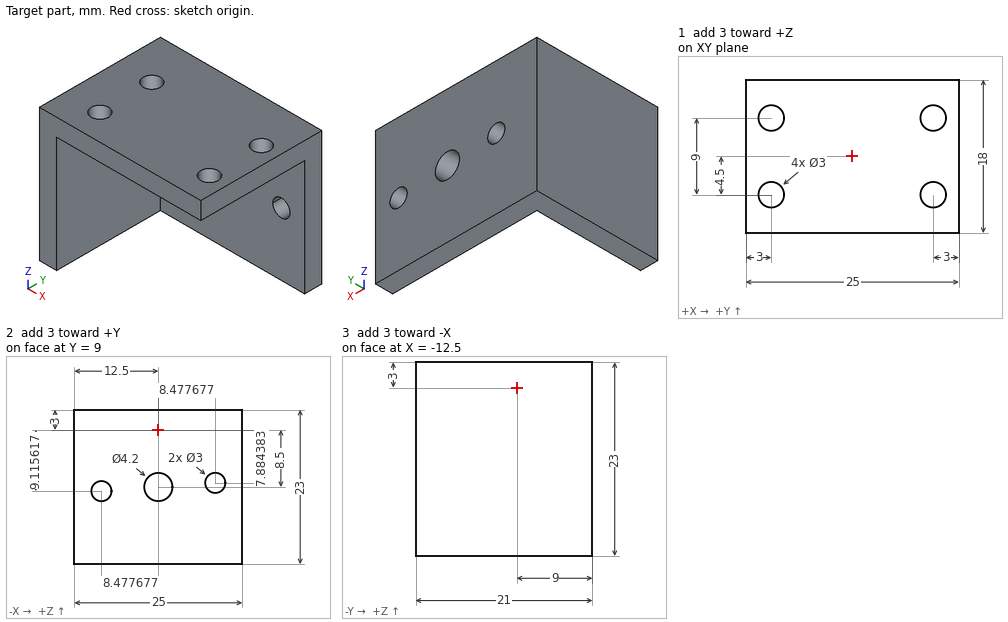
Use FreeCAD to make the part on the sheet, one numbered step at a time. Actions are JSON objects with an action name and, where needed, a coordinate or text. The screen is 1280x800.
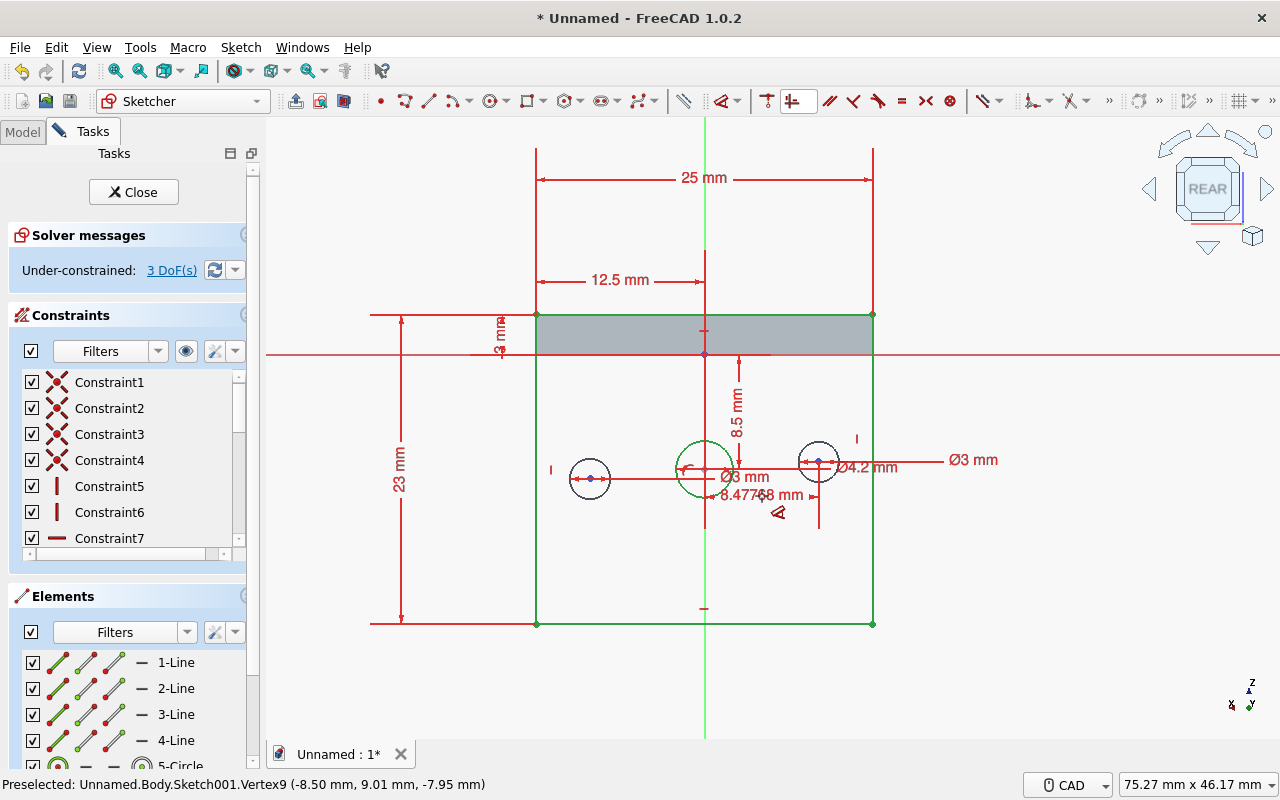
{"action": "left_click", "coordinate": [819, 462]}
{"action": "left_click", "coordinate": [853, 408]}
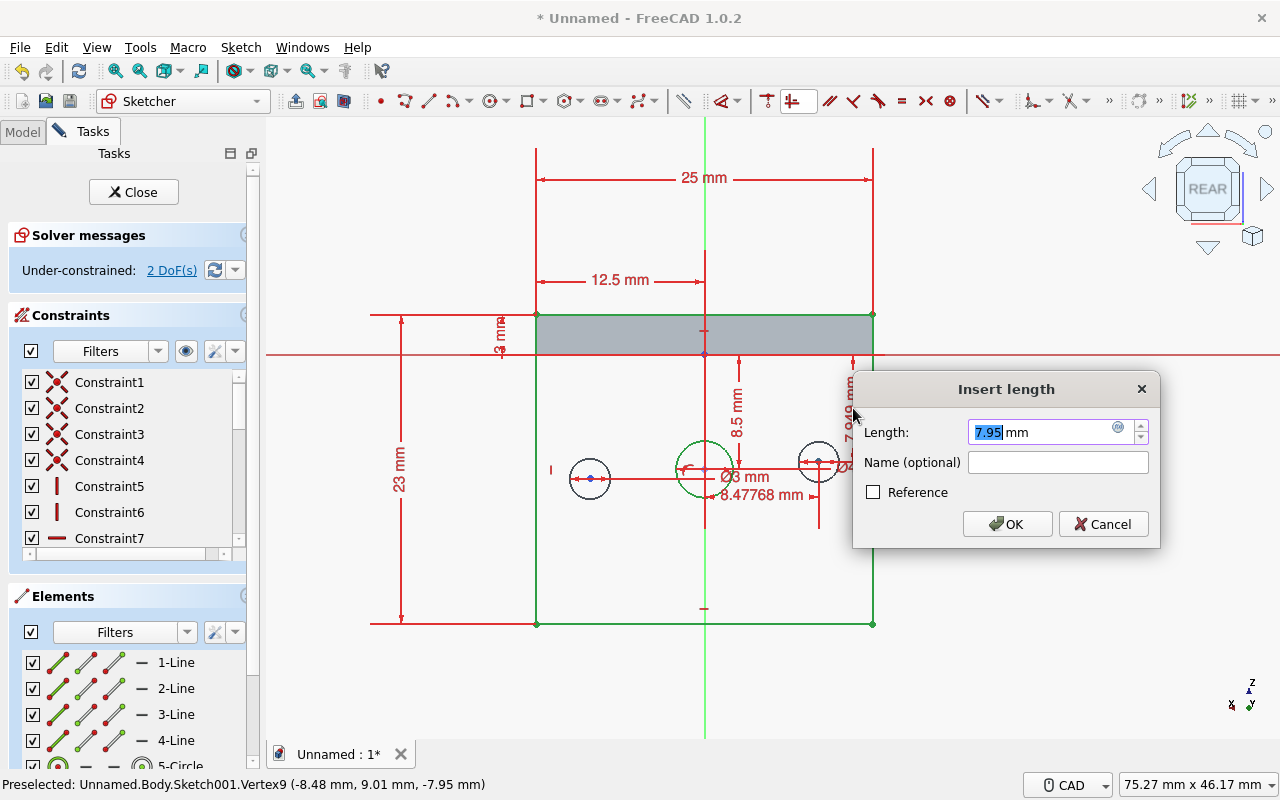
{"action": "type", "text": "7.884383"}
{"action": "key", "text": "Return"}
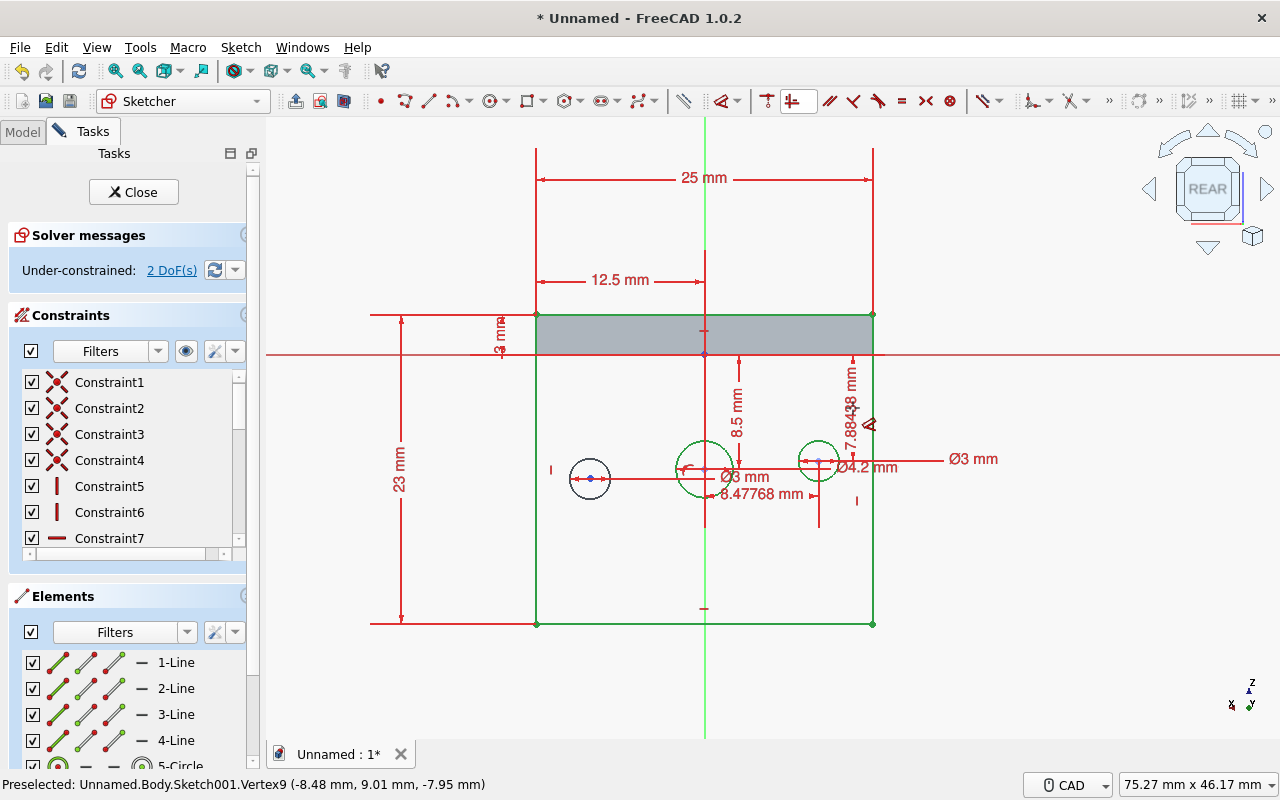
{"action": "left_click", "coordinate": [590, 479]}
{"action": "left_click", "coordinate": [647, 513]}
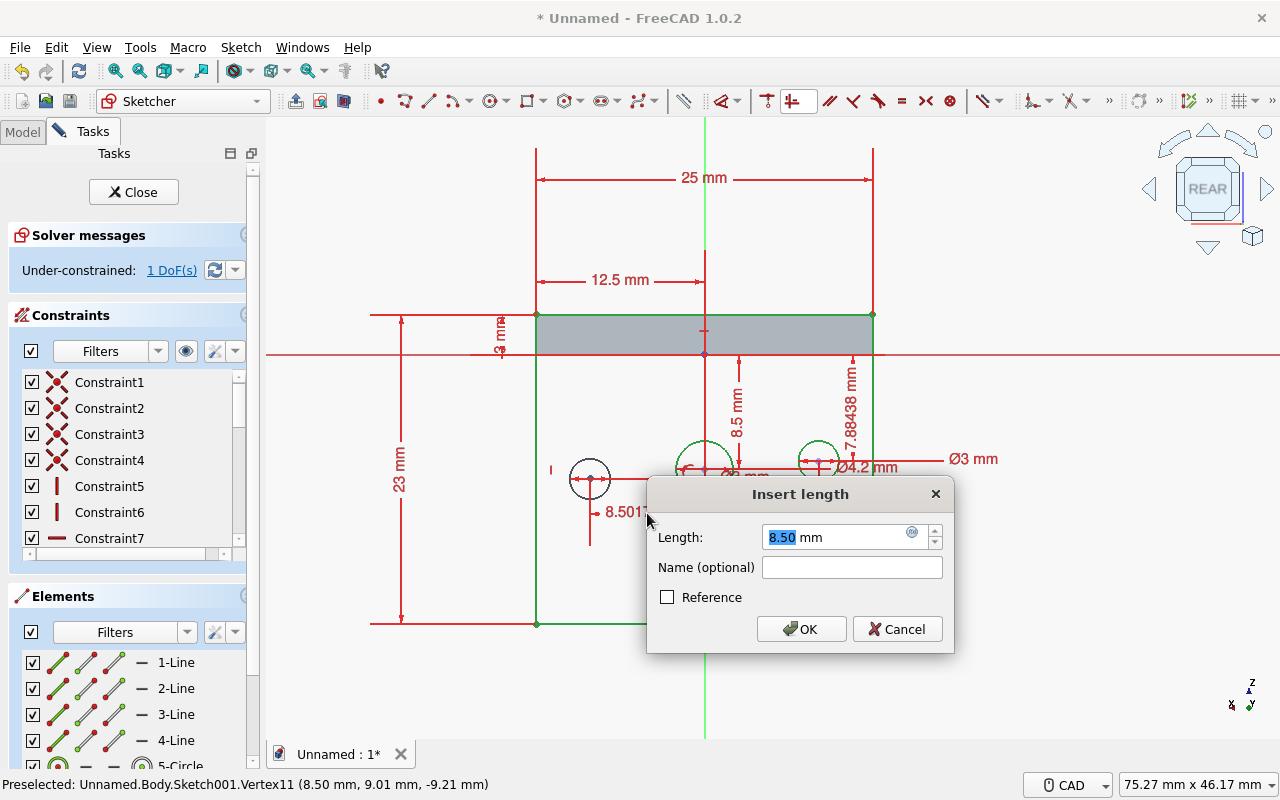
{"action": "type", "text": "8.477677"}
{"action": "key", "text": "Return"}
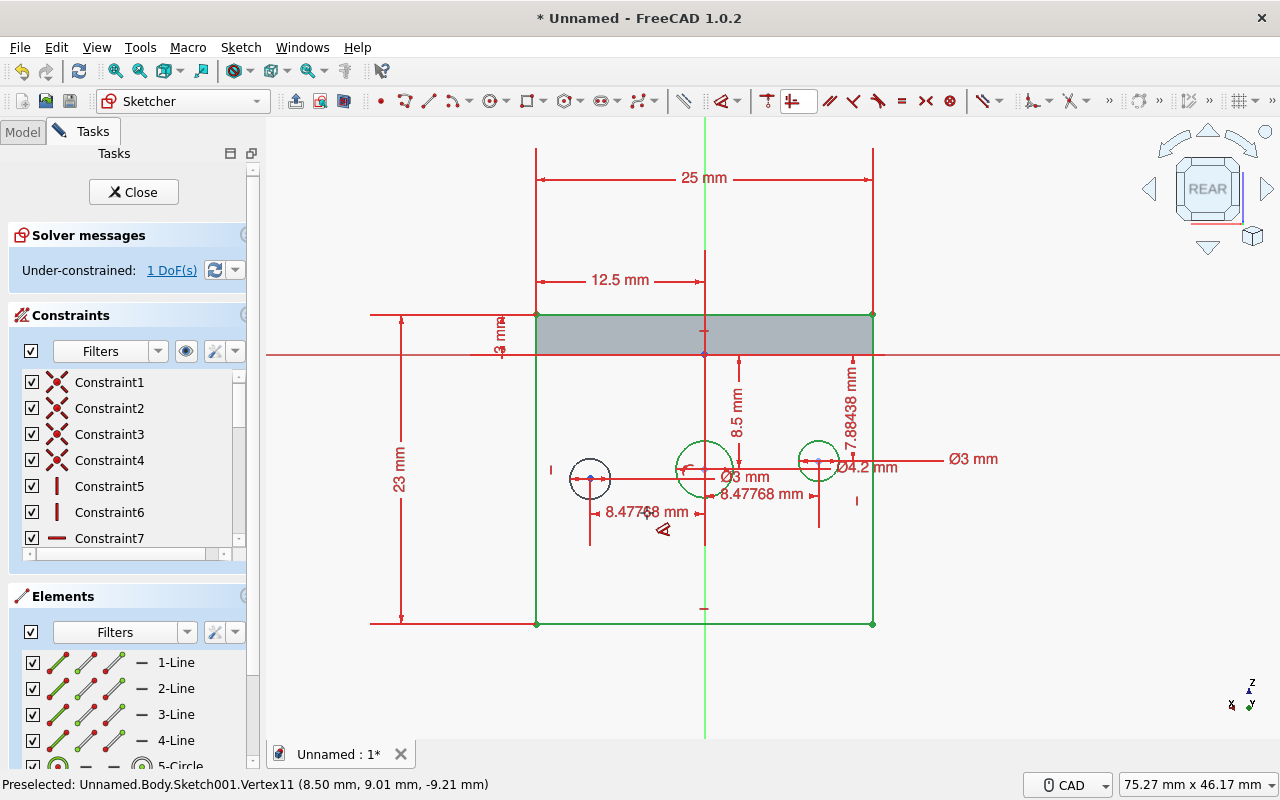
{"action": "left_click", "coordinate": [590, 479]}
{"action": "left_click", "coordinate": [556, 417]}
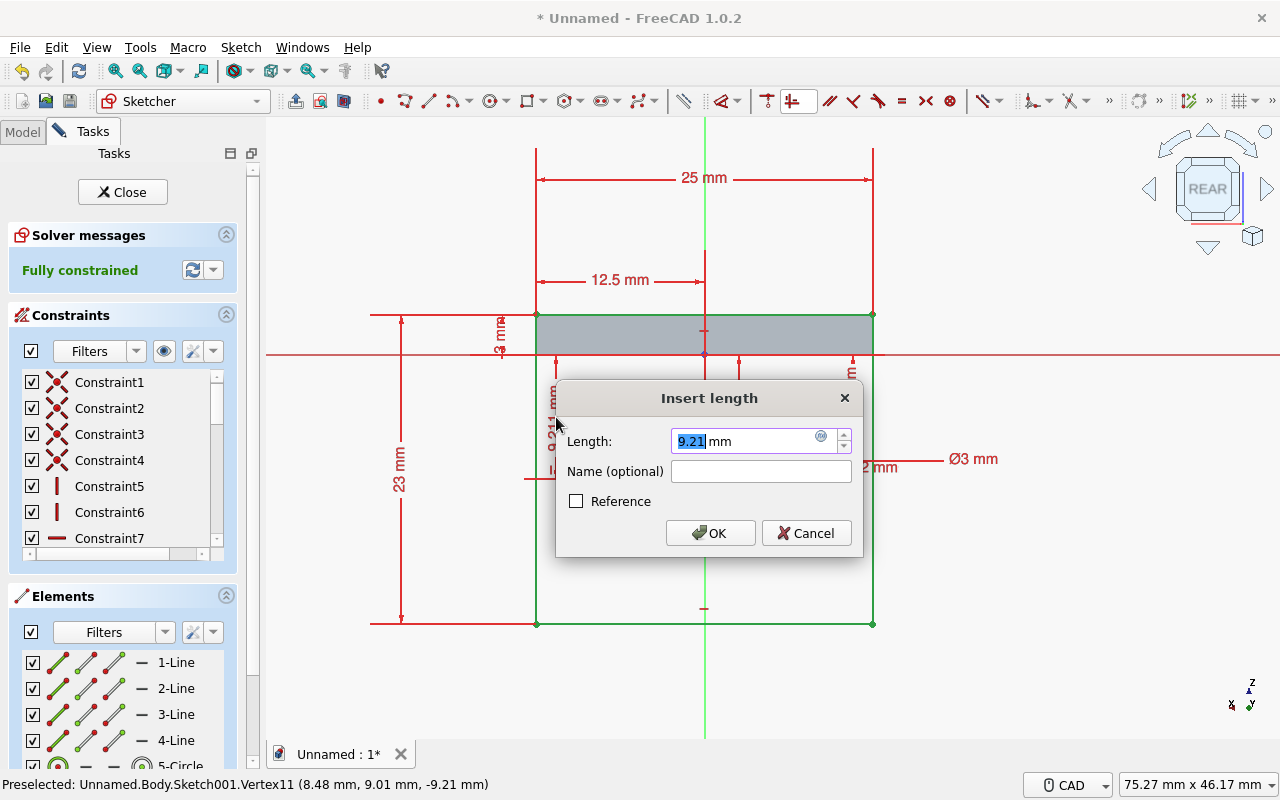
{"action": "type", "text": "9.115617"}
{"action": "key", "text": "Return"}
{"action": "key", "text": "Escape"}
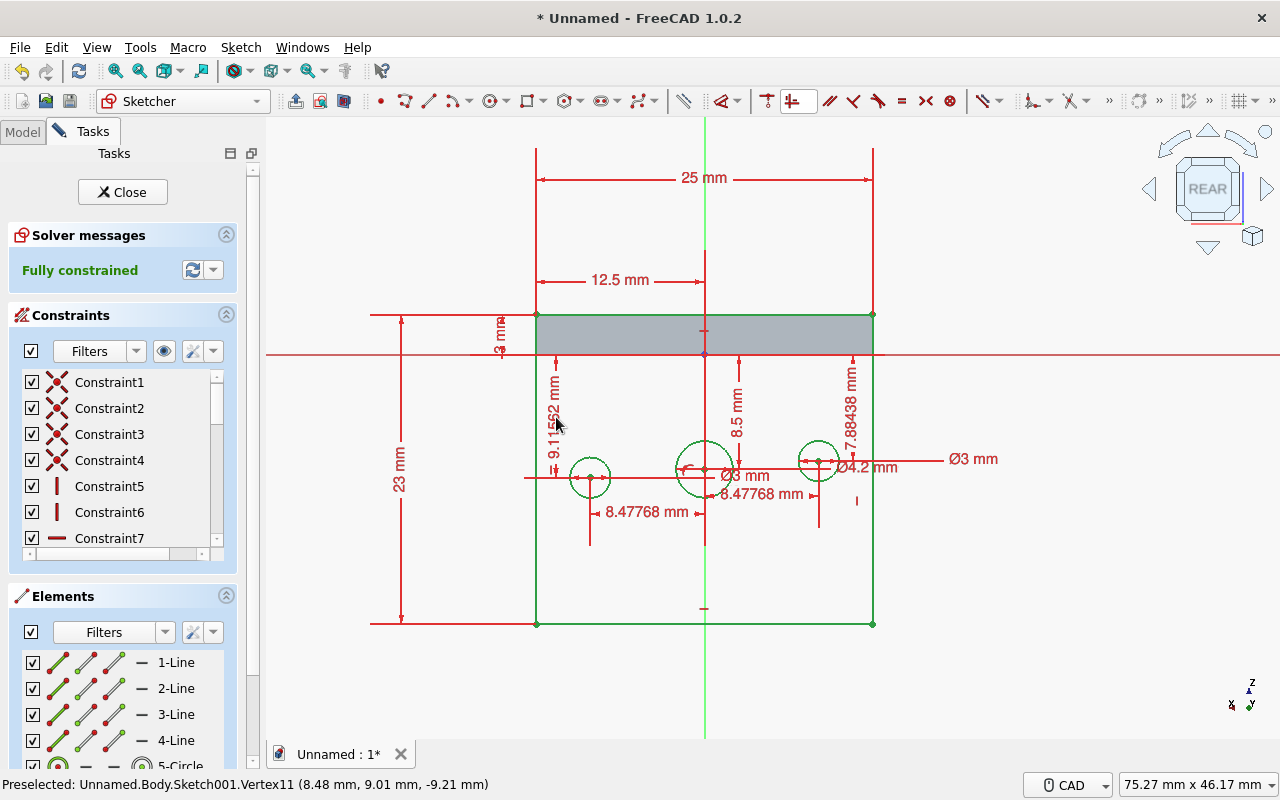
{"action": "left_click", "coordinate": [123, 192]}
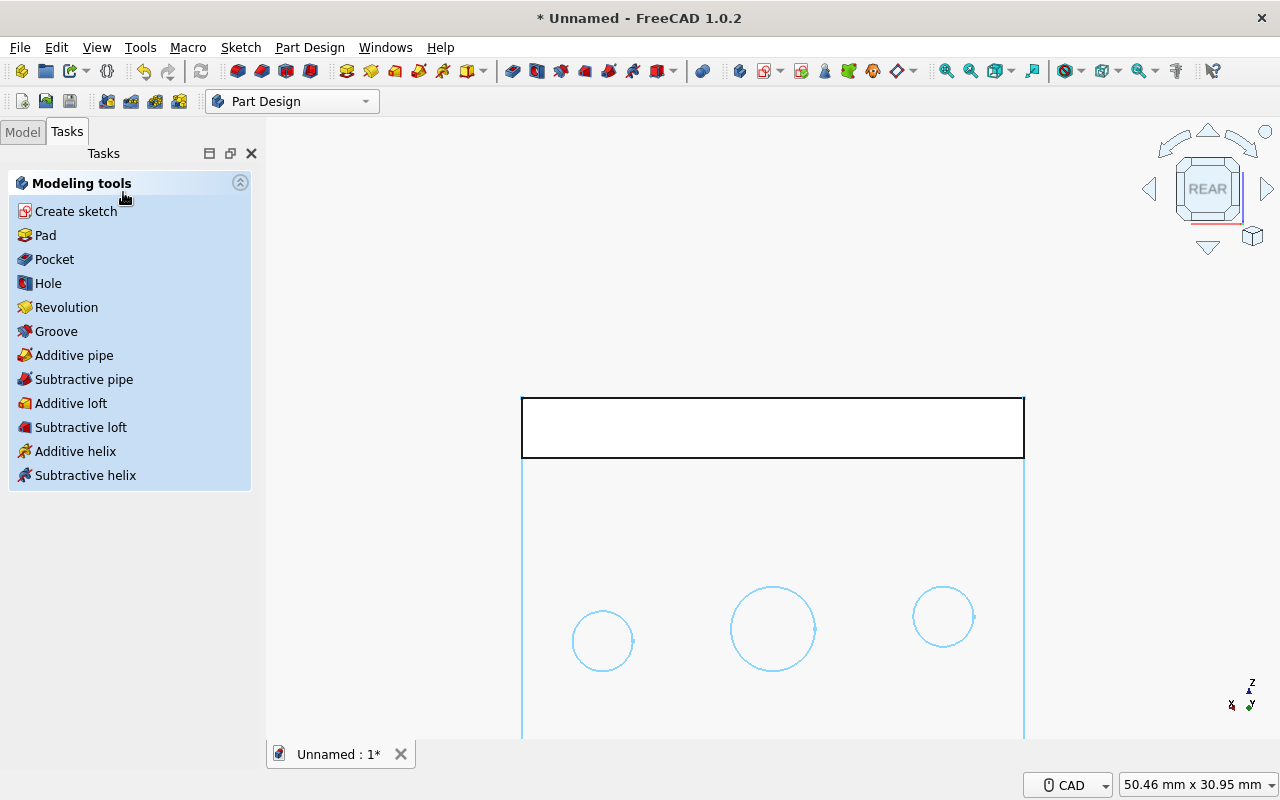
{"action": "left_click", "coordinate": [348, 72]}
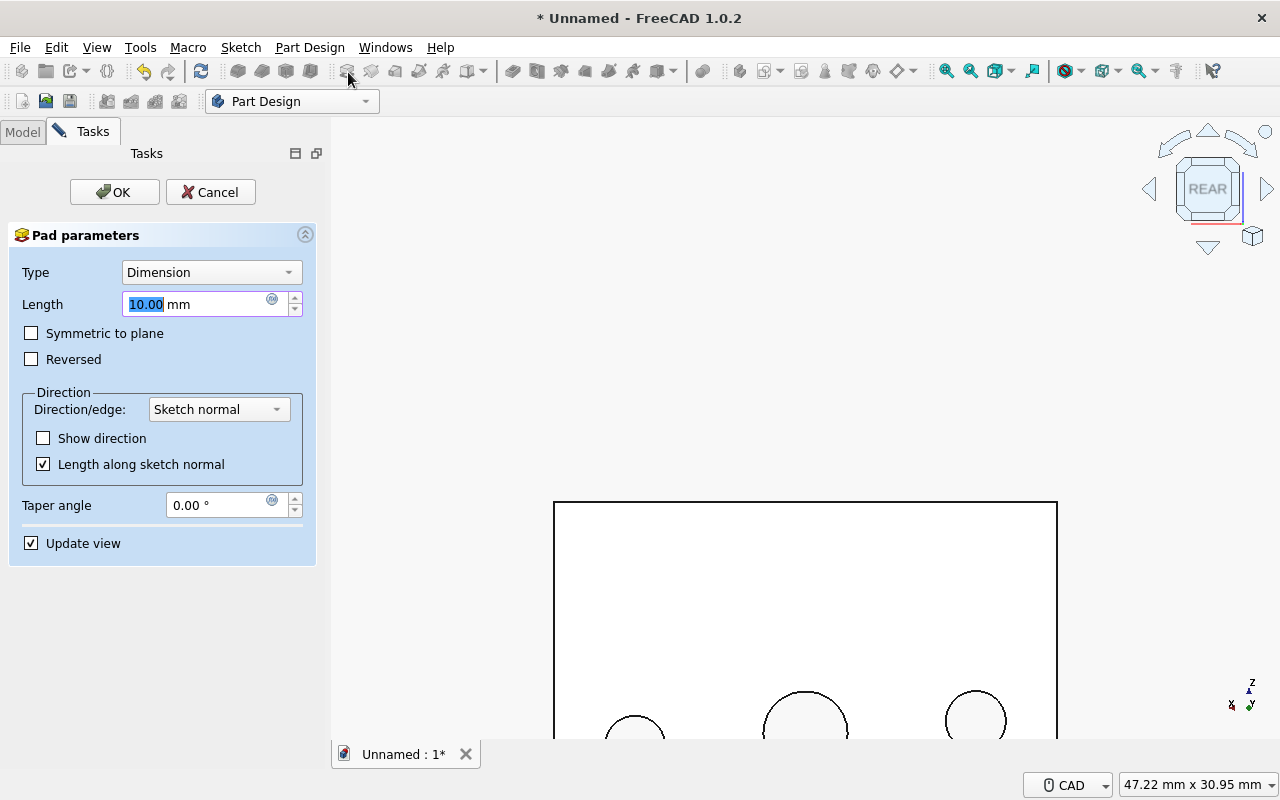
{"action": "type", "text": "3"}
{"action": "key", "text": "Tab"}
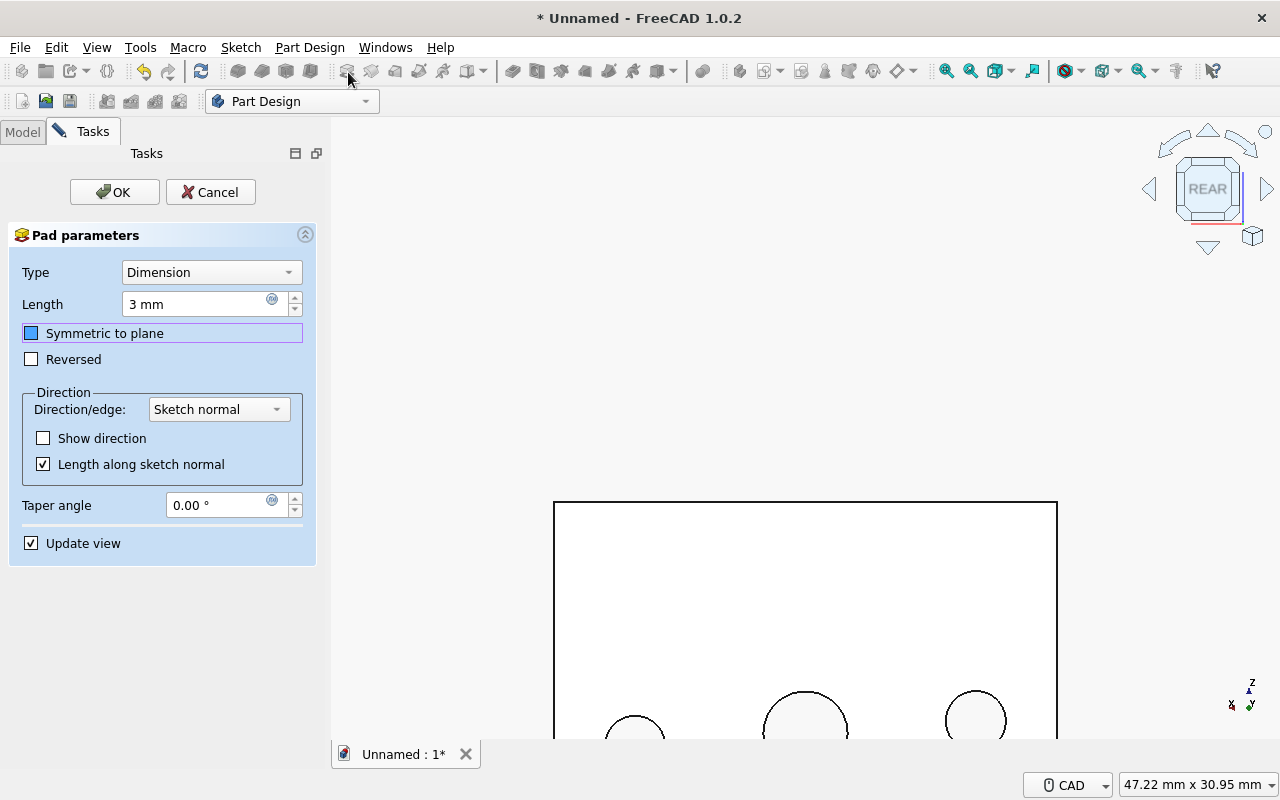
{"action": "left_click", "coordinate": [115, 192]}